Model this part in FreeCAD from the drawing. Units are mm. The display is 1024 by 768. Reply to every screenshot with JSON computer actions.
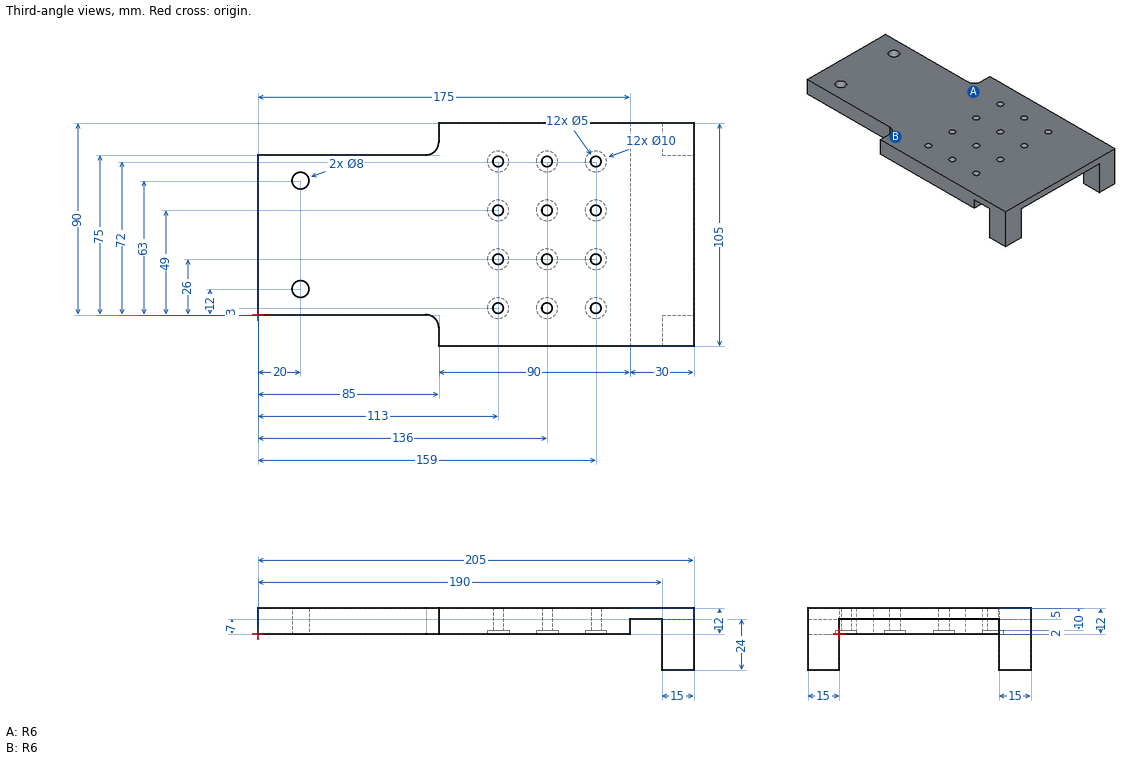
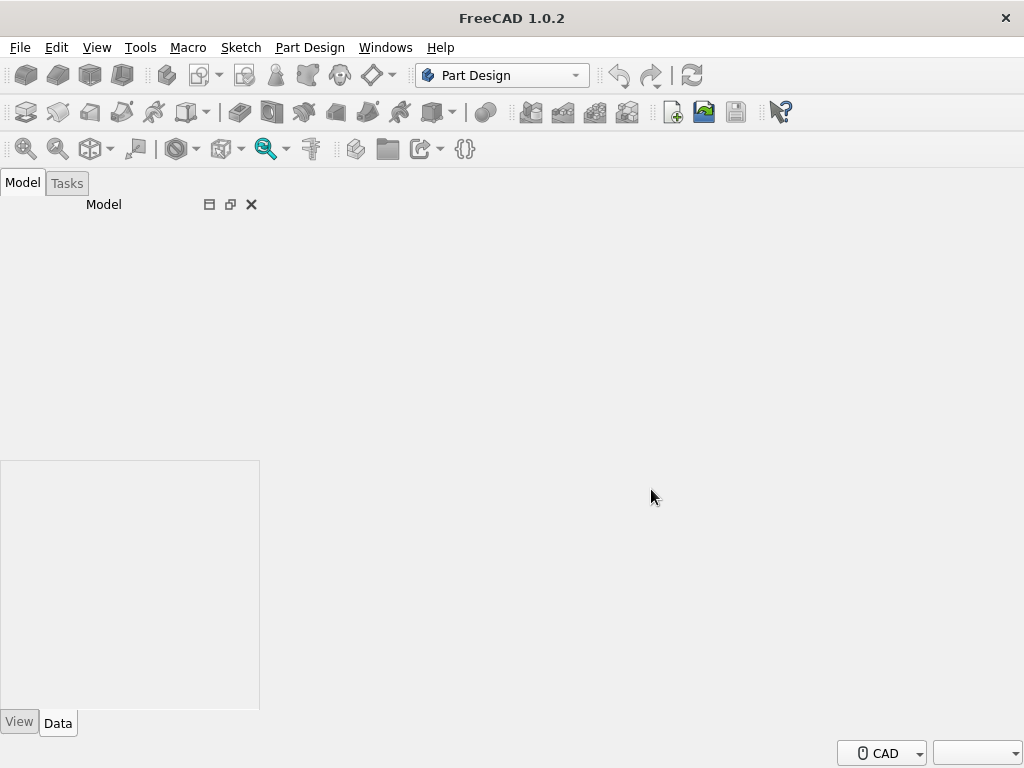
{"action": "left_click", "coordinate": [672, 112]}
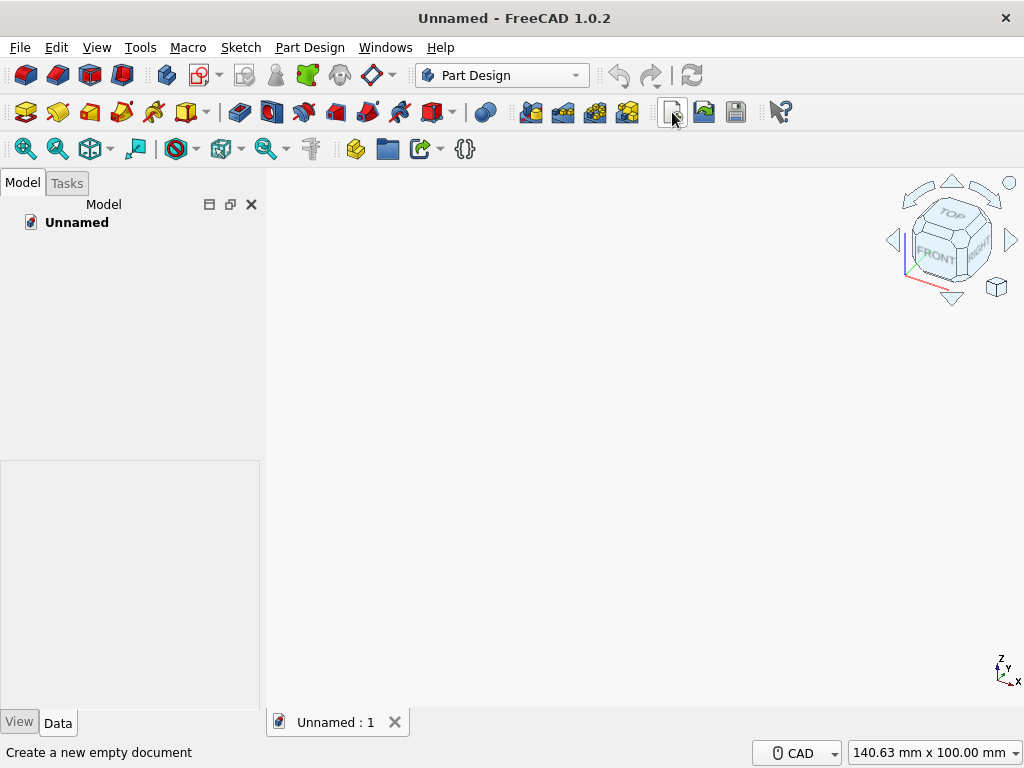
{"action": "left_click", "coordinate": [200, 76]}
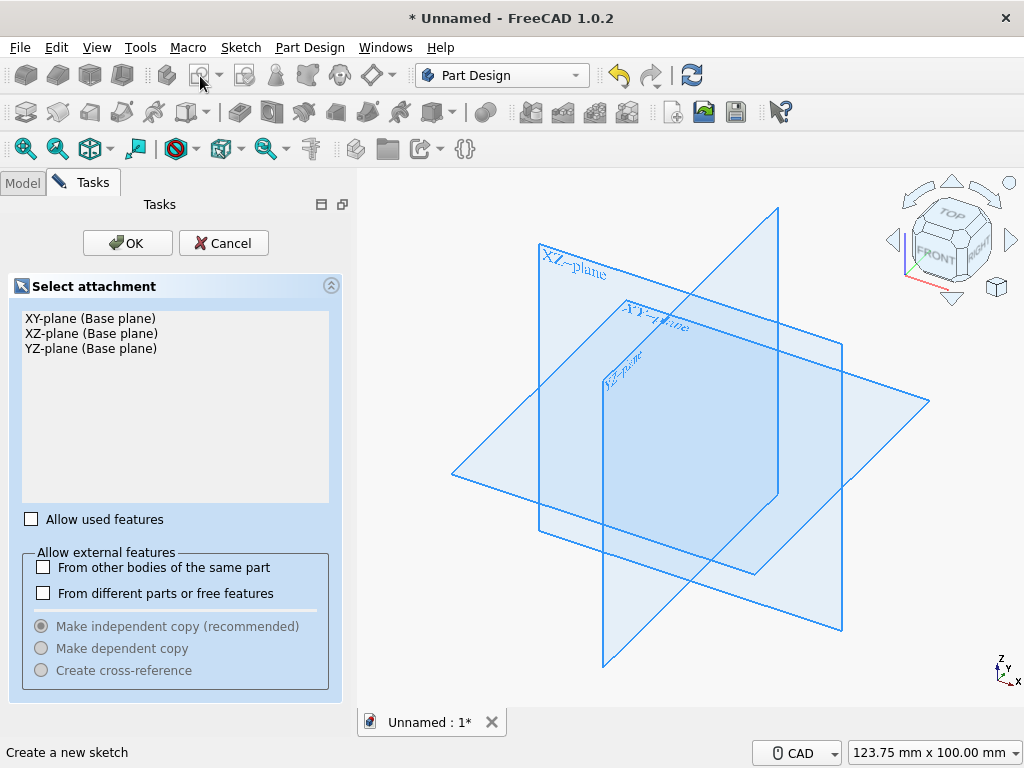
{"action": "left_click", "coordinate": [82, 318]}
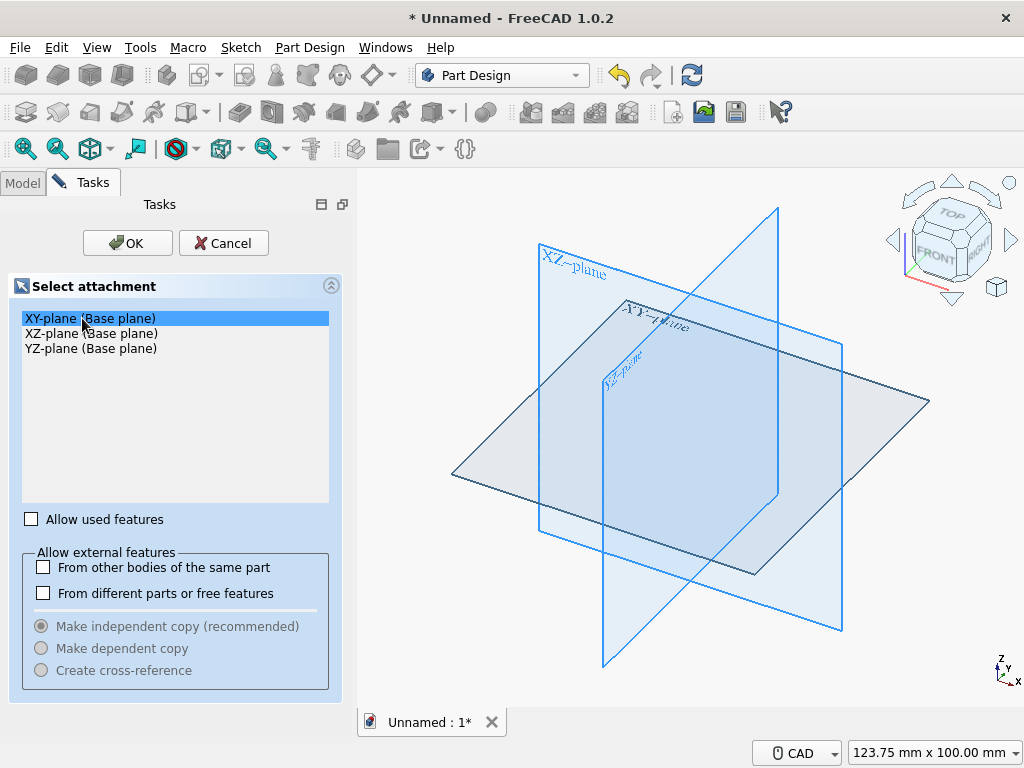
{"action": "left_click", "coordinate": [128, 243]}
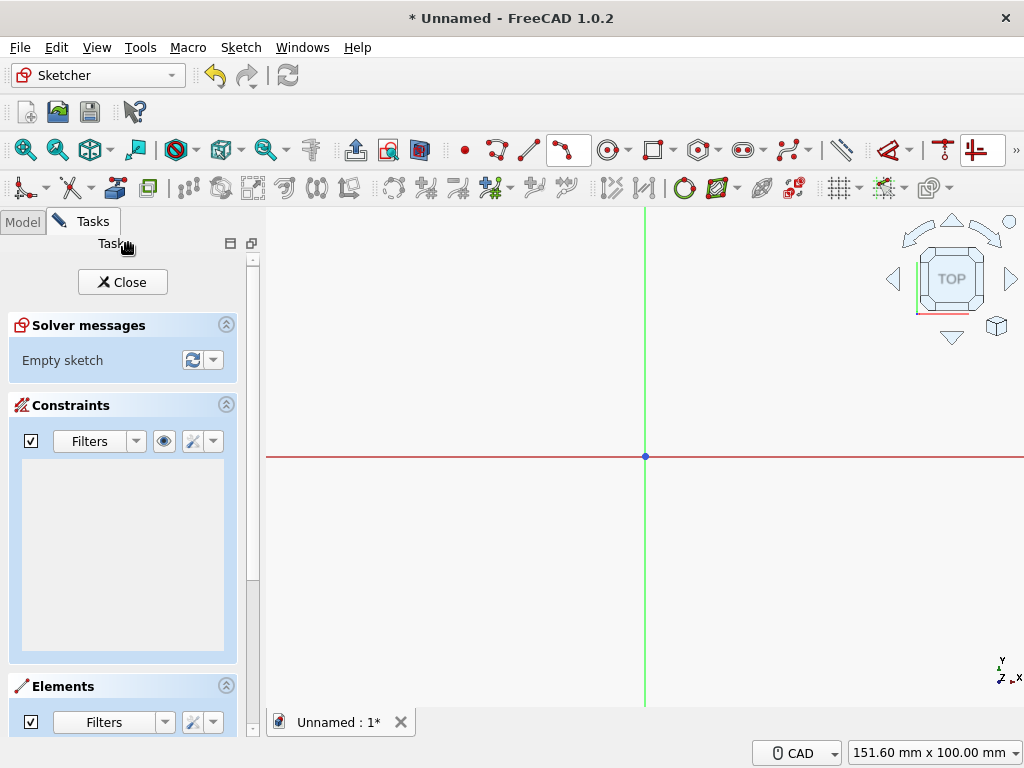
{"action": "scroll", "coordinate": [294, 679], "scroll_direction": "down", "scroll_amount": 2}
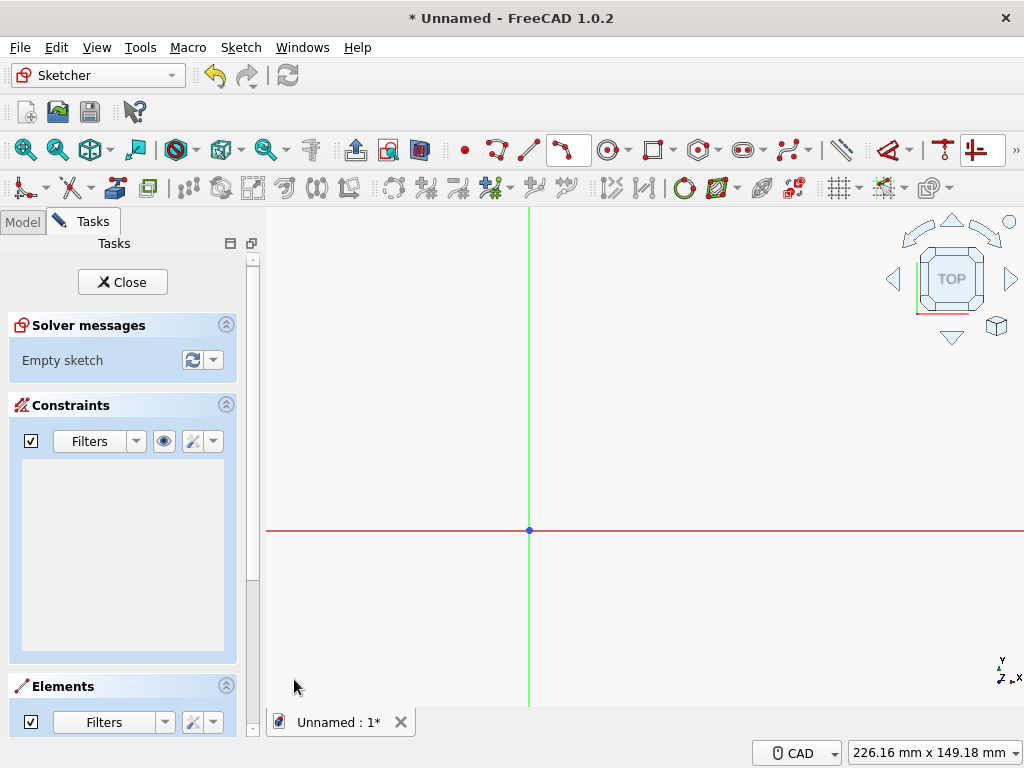
{"action": "left_click", "coordinate": [654, 150]}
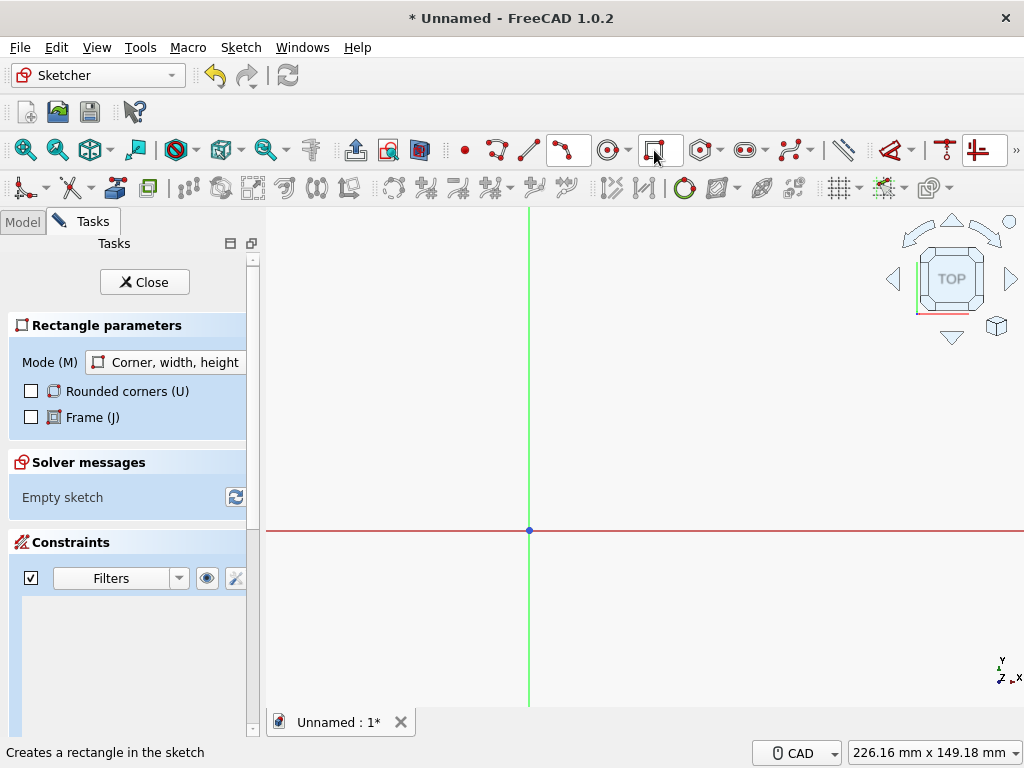
{"action": "left_click", "coordinate": [529, 531]}
{"action": "mouse_move", "coordinate": [814, 279]}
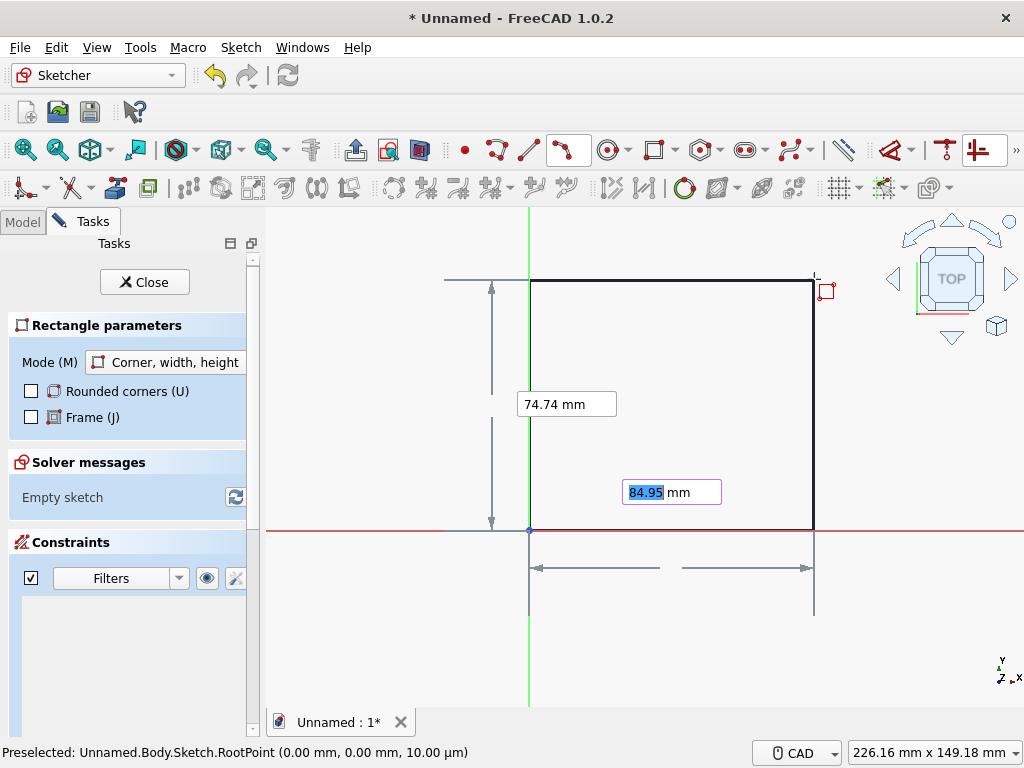
{"action": "type", "text": "85"}
{"action": "key", "text": "Tab"}
{"action": "type", "text": "75"}
{"action": "key", "text": "Return"}
{"action": "key", "text": "Escape"}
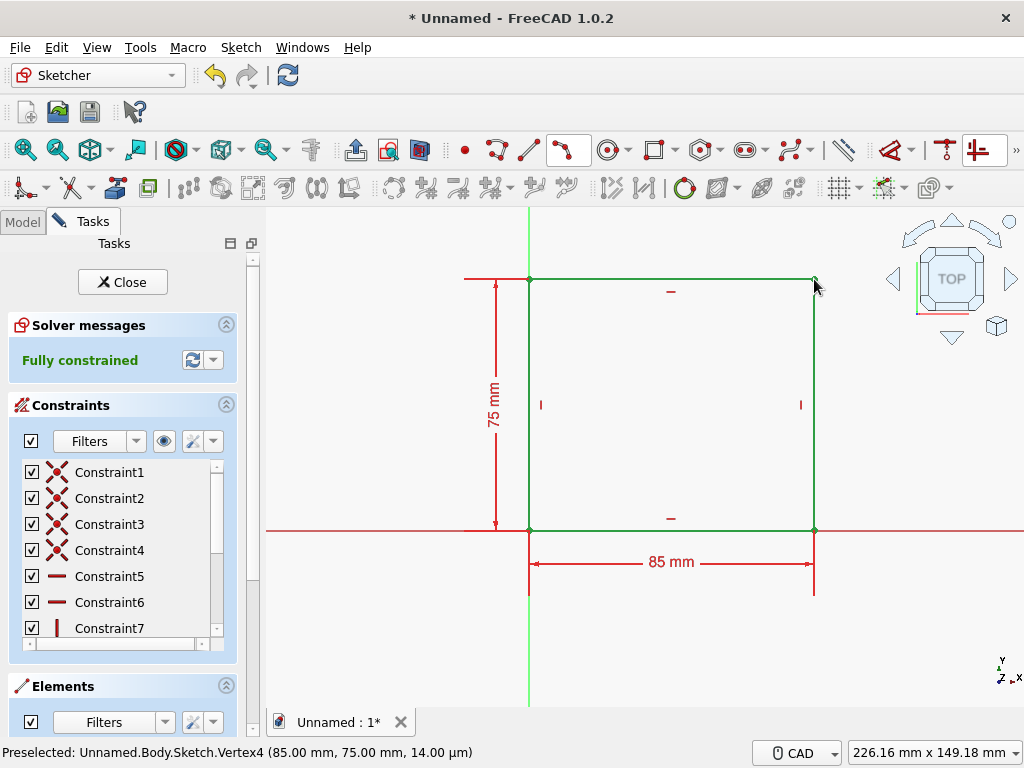
{"action": "left_click", "coordinate": [123, 282]}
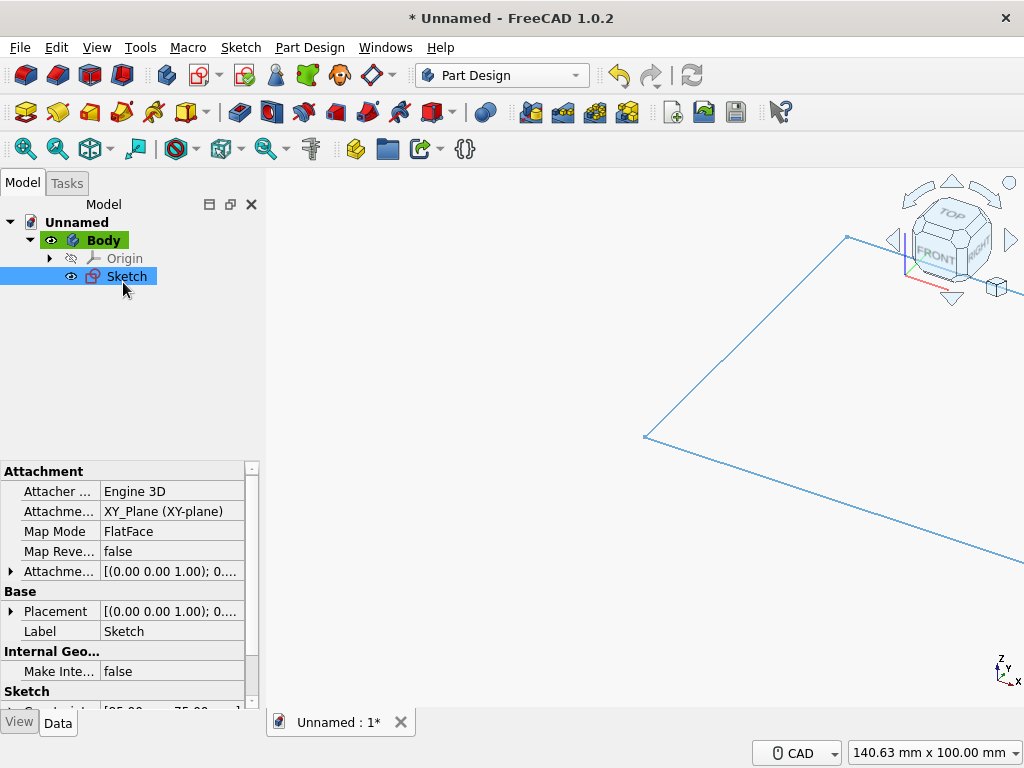
{"action": "left_click", "coordinate": [26, 112]}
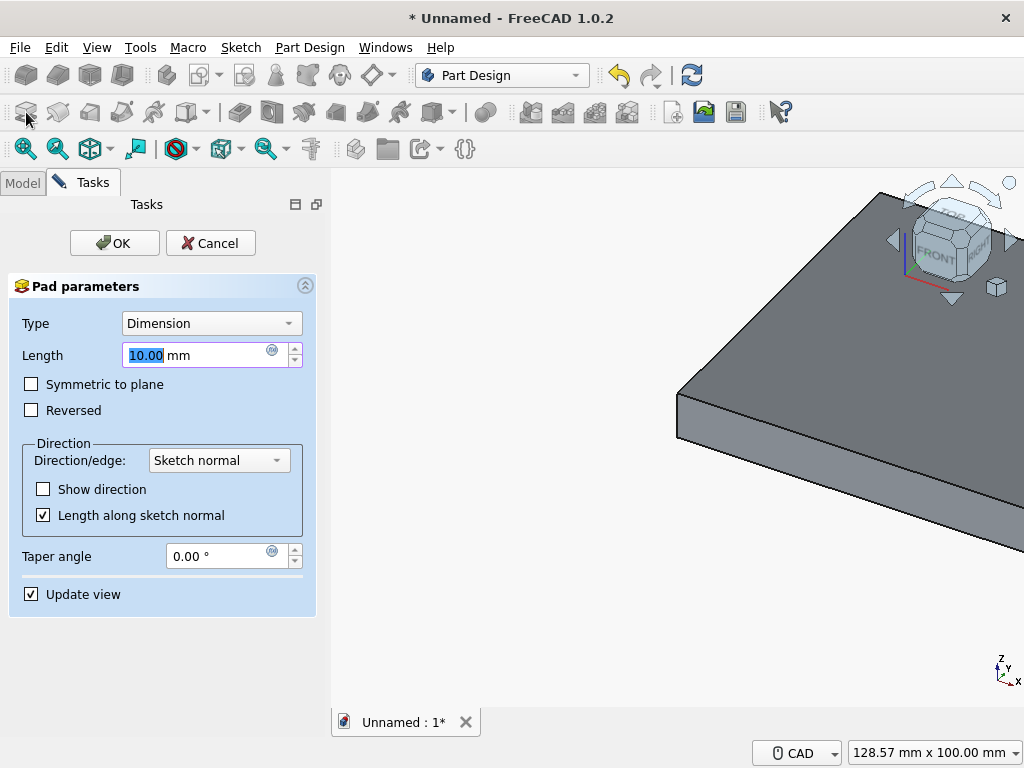
{"action": "type", "text": "12"}
{"action": "key", "text": "Tab"}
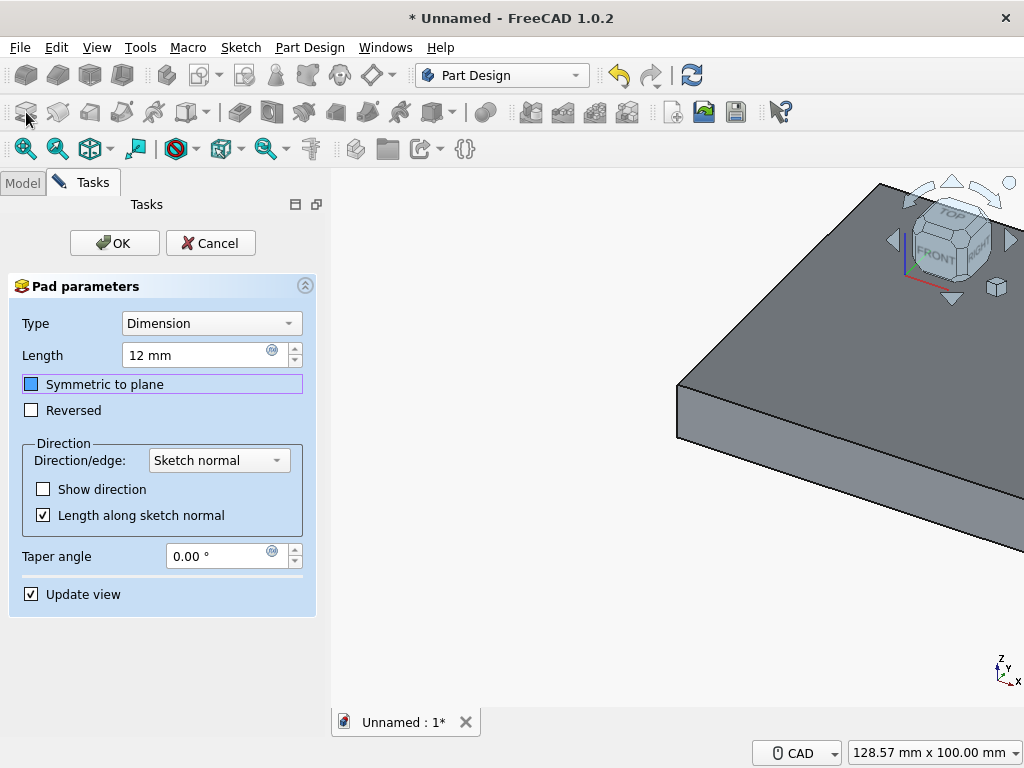
{"action": "left_click", "coordinate": [115, 243]}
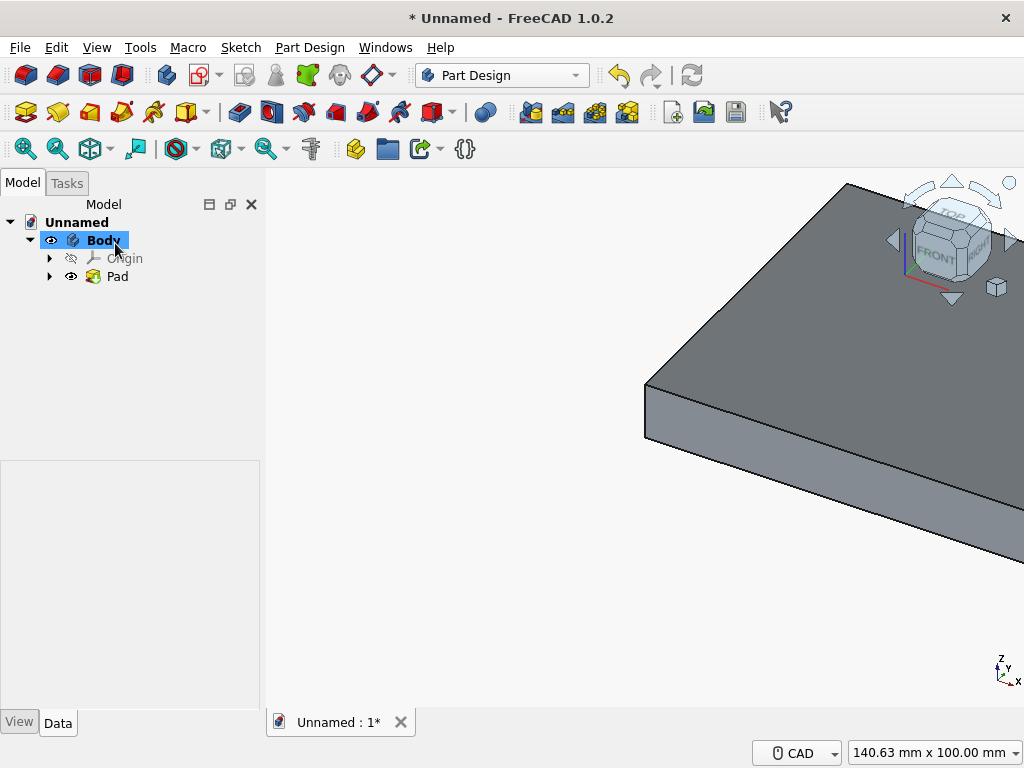
{"action": "left_click", "coordinate": [26, 150]}